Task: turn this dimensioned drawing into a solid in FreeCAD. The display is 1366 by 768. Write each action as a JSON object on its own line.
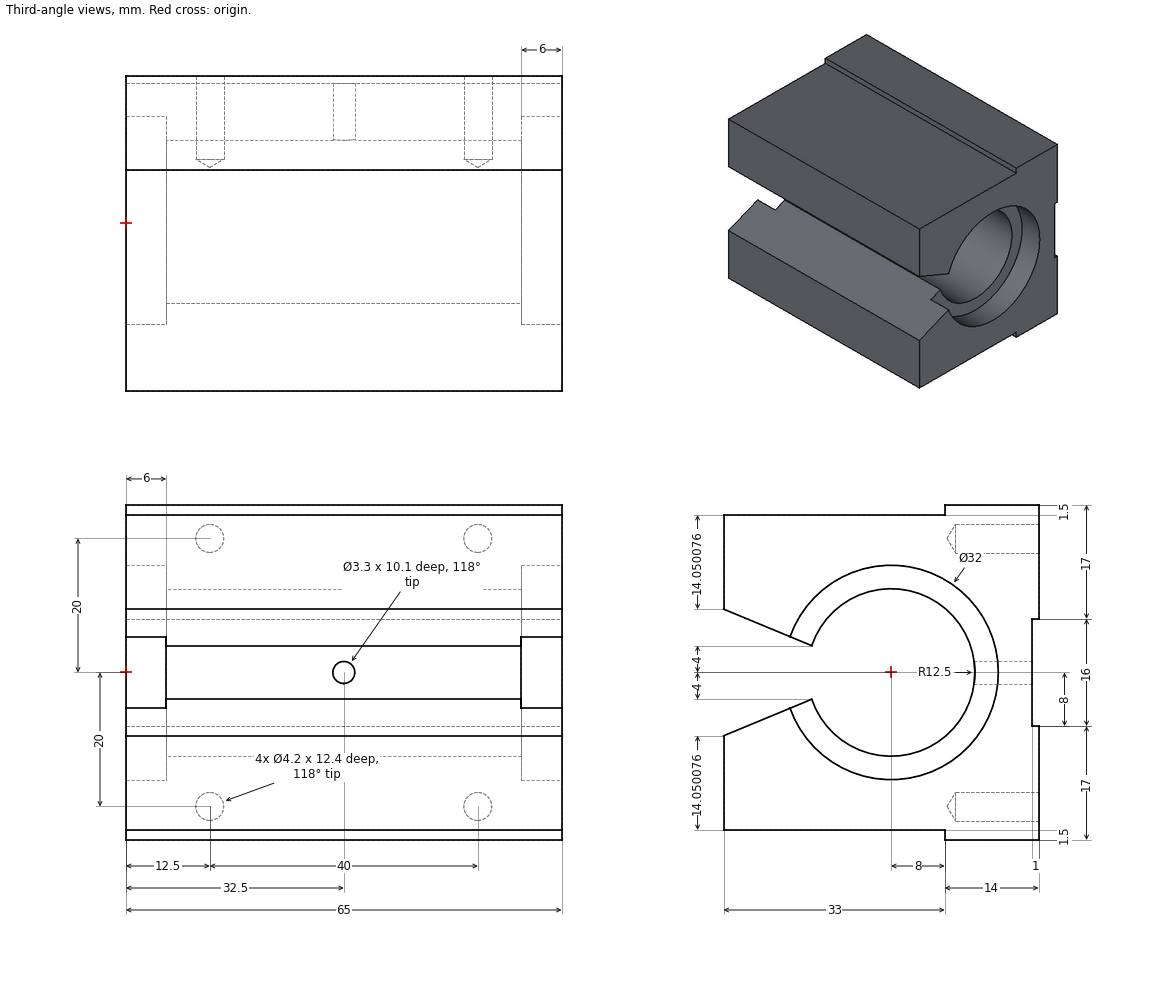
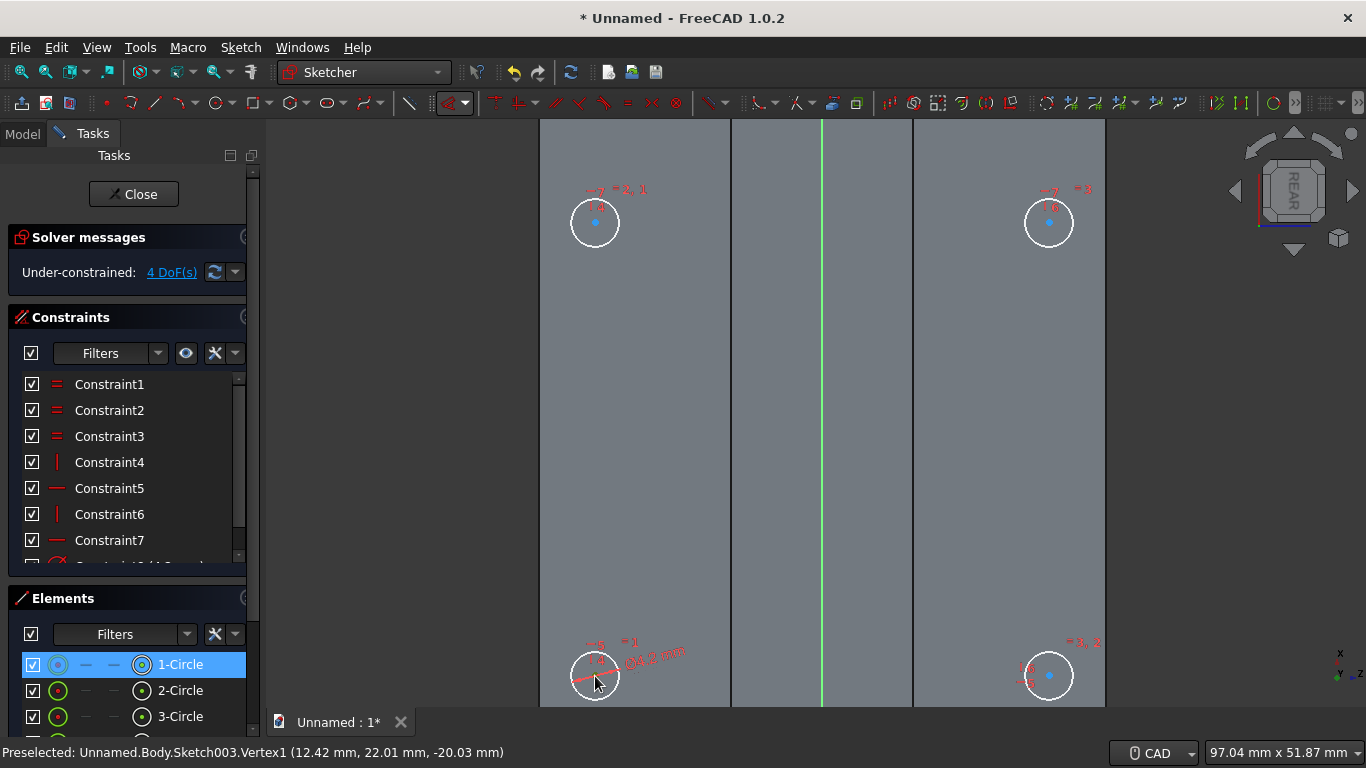
{"action": "key", "text": "l"}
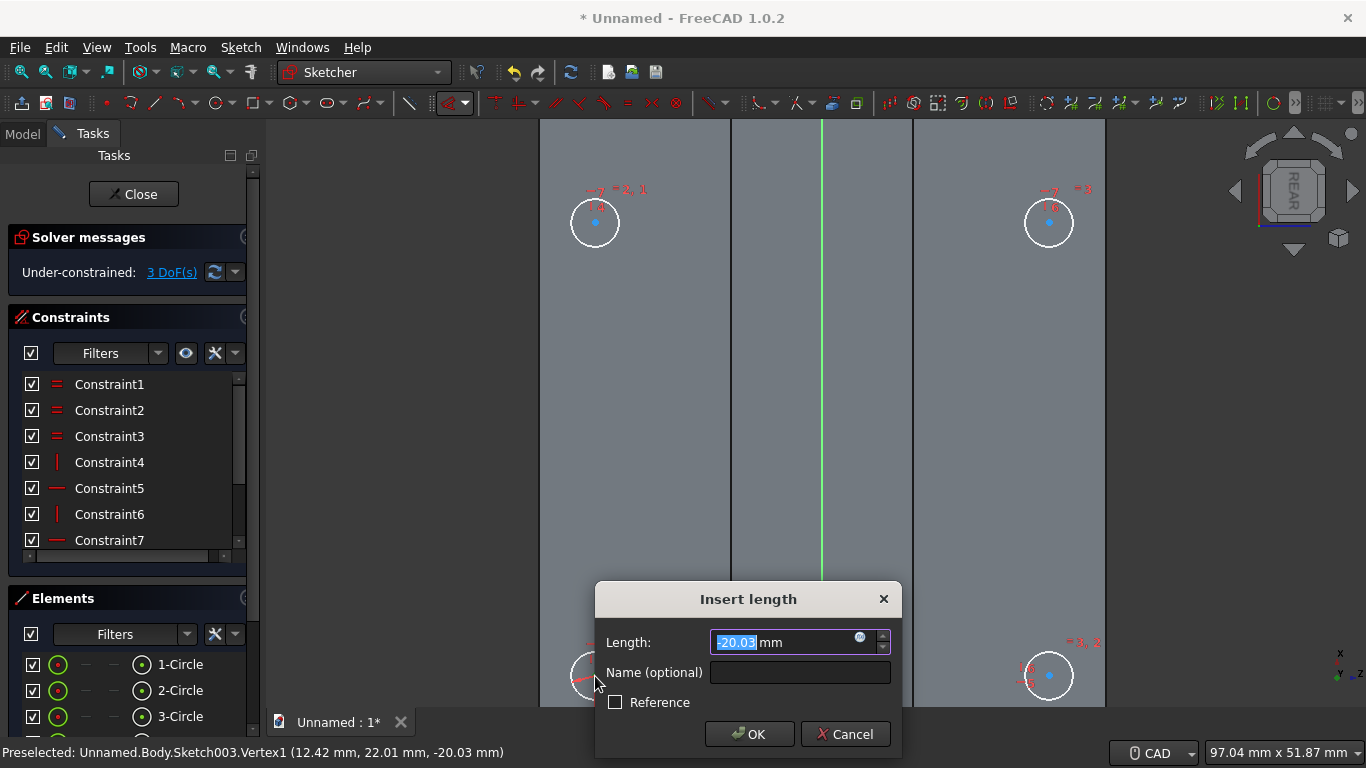
{"action": "type", "text": "-20"}
{"action": "key", "text": "Return"}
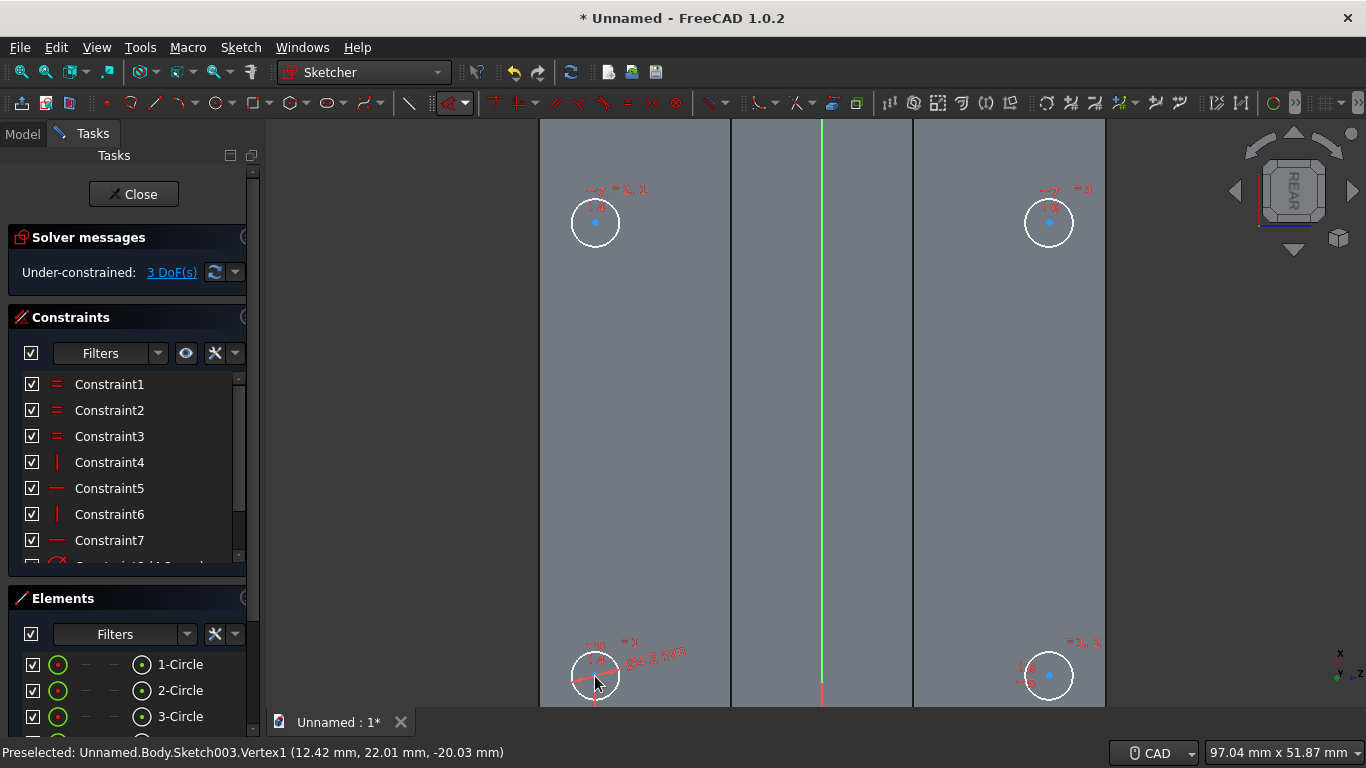
{"action": "left_click", "coordinate": [1049, 676]}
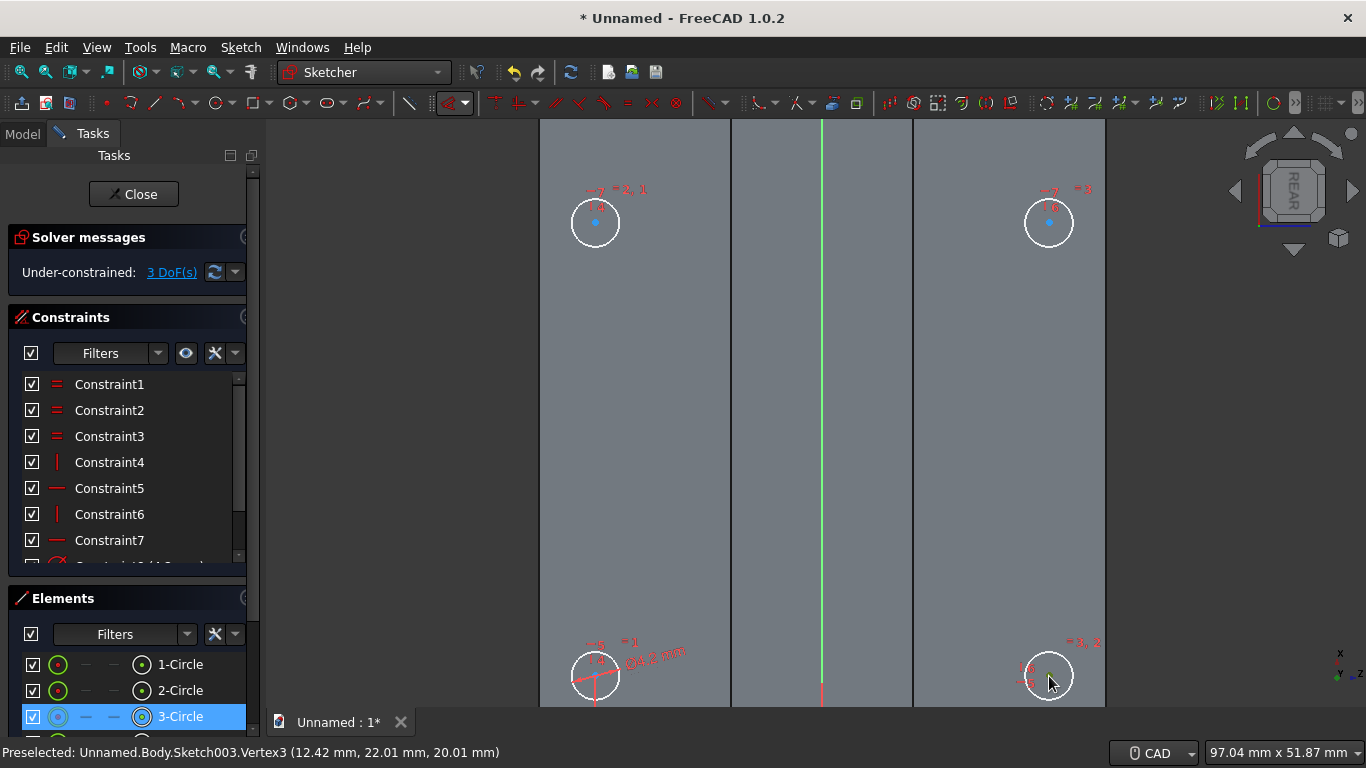
{"action": "left_click", "coordinate": [468, 104]}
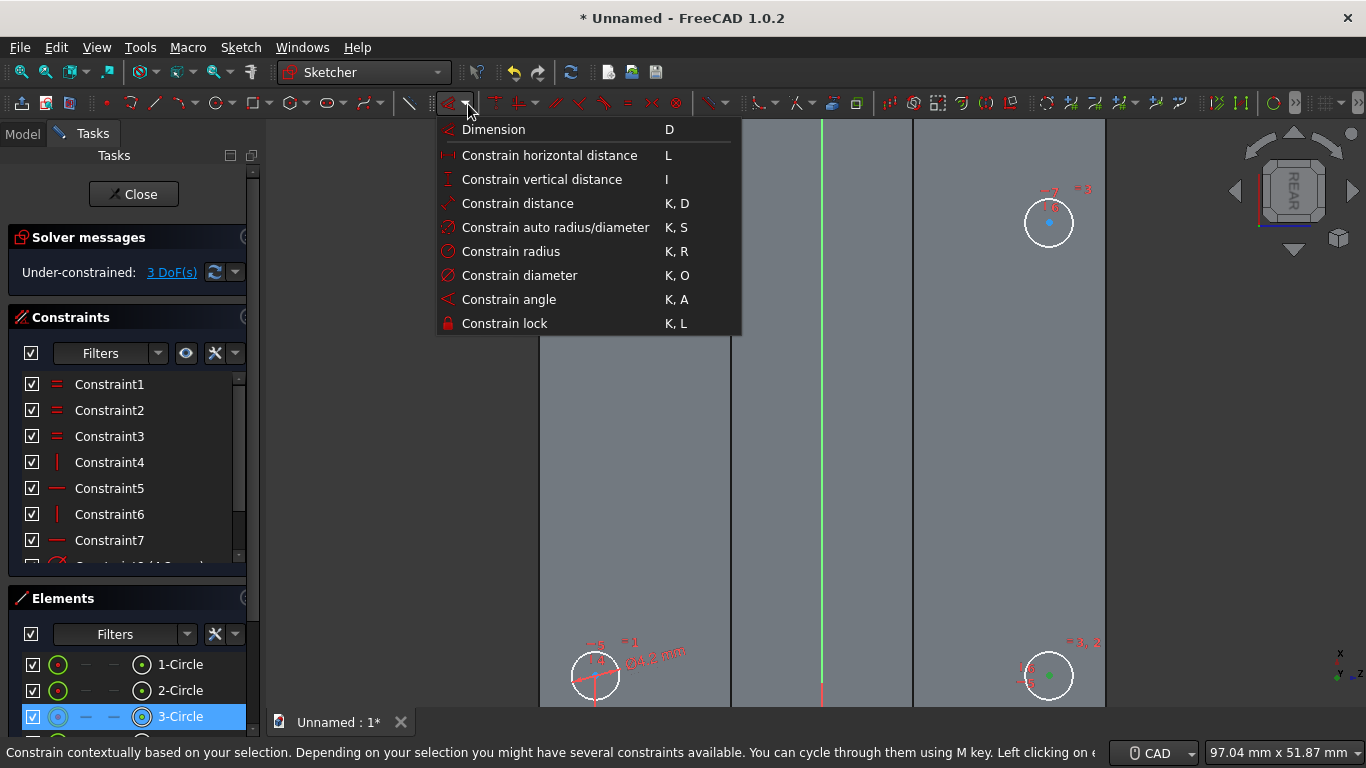
{"action": "left_click", "coordinate": [589, 155]}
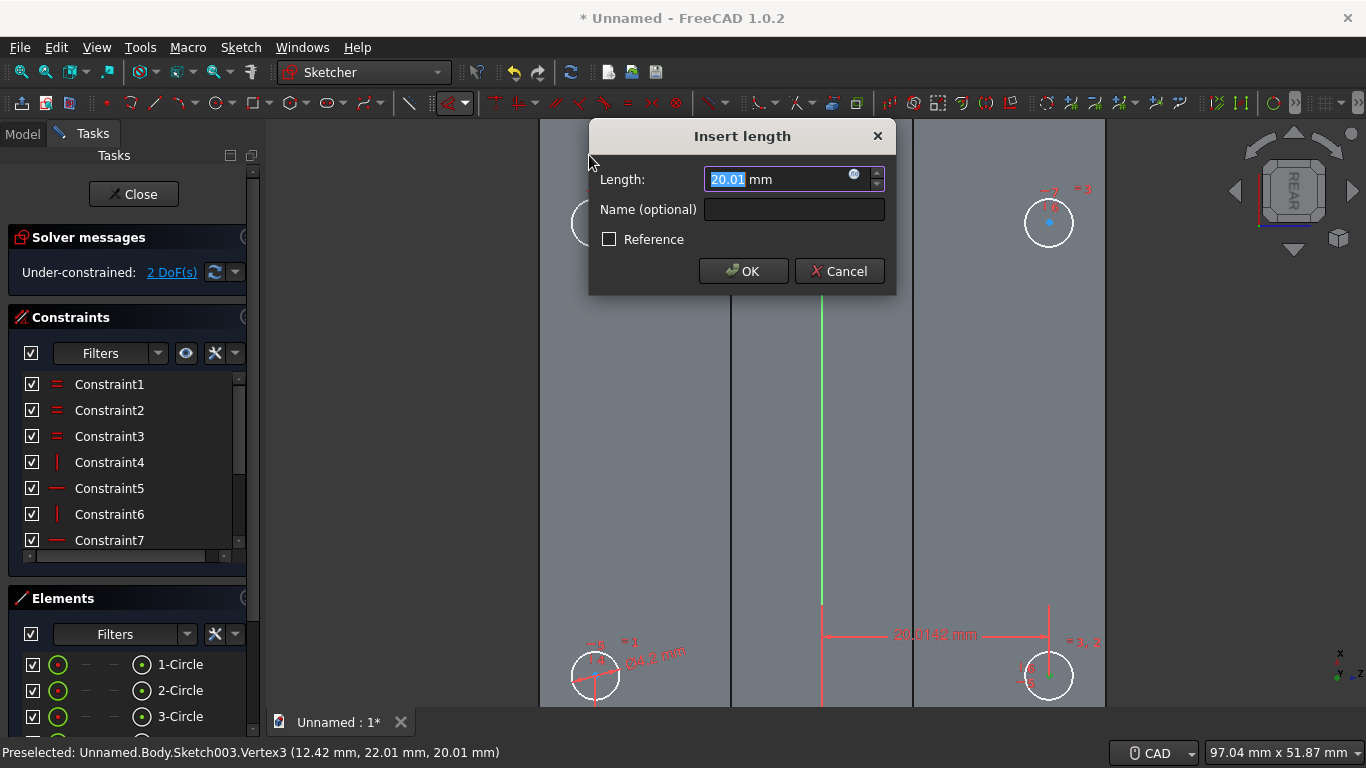
{"action": "type", "text": "20"}
{"action": "key", "text": "Return"}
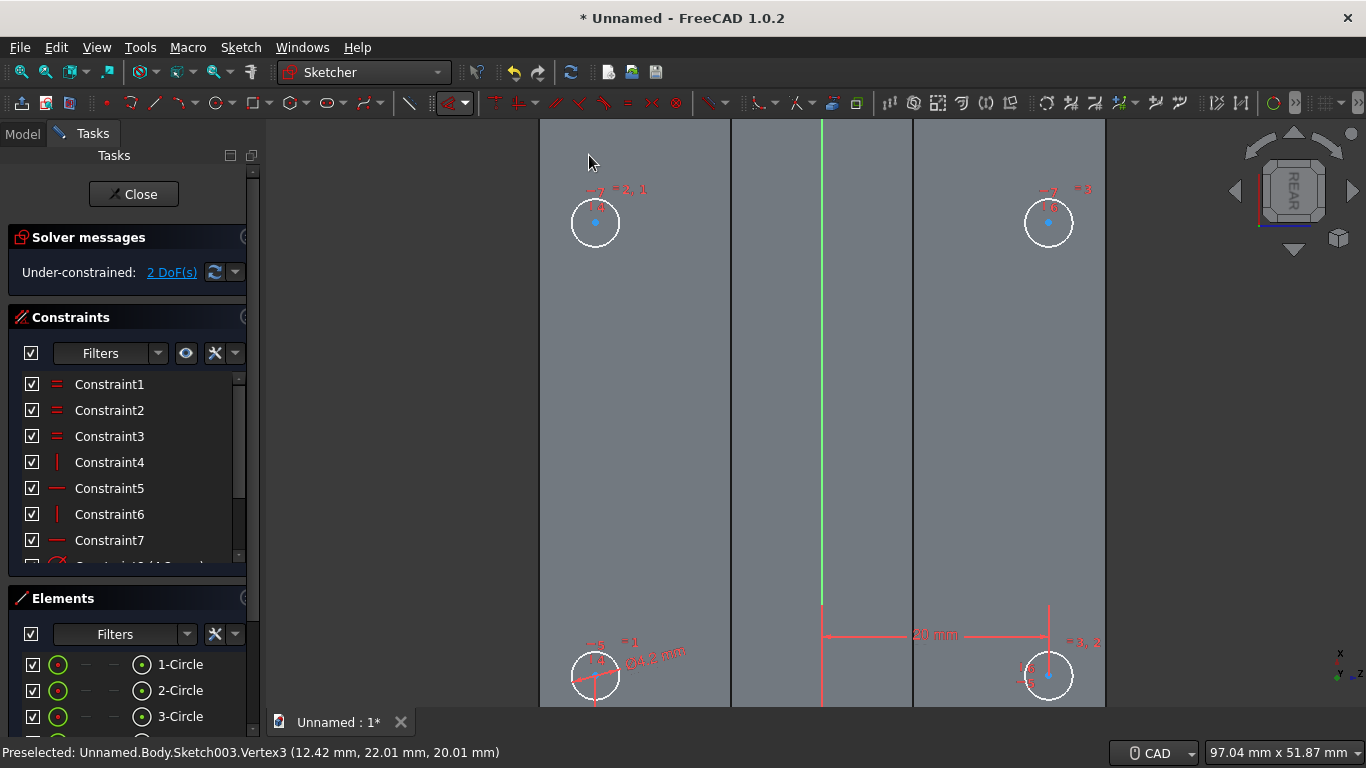
{"action": "left_click", "coordinate": [595, 676]}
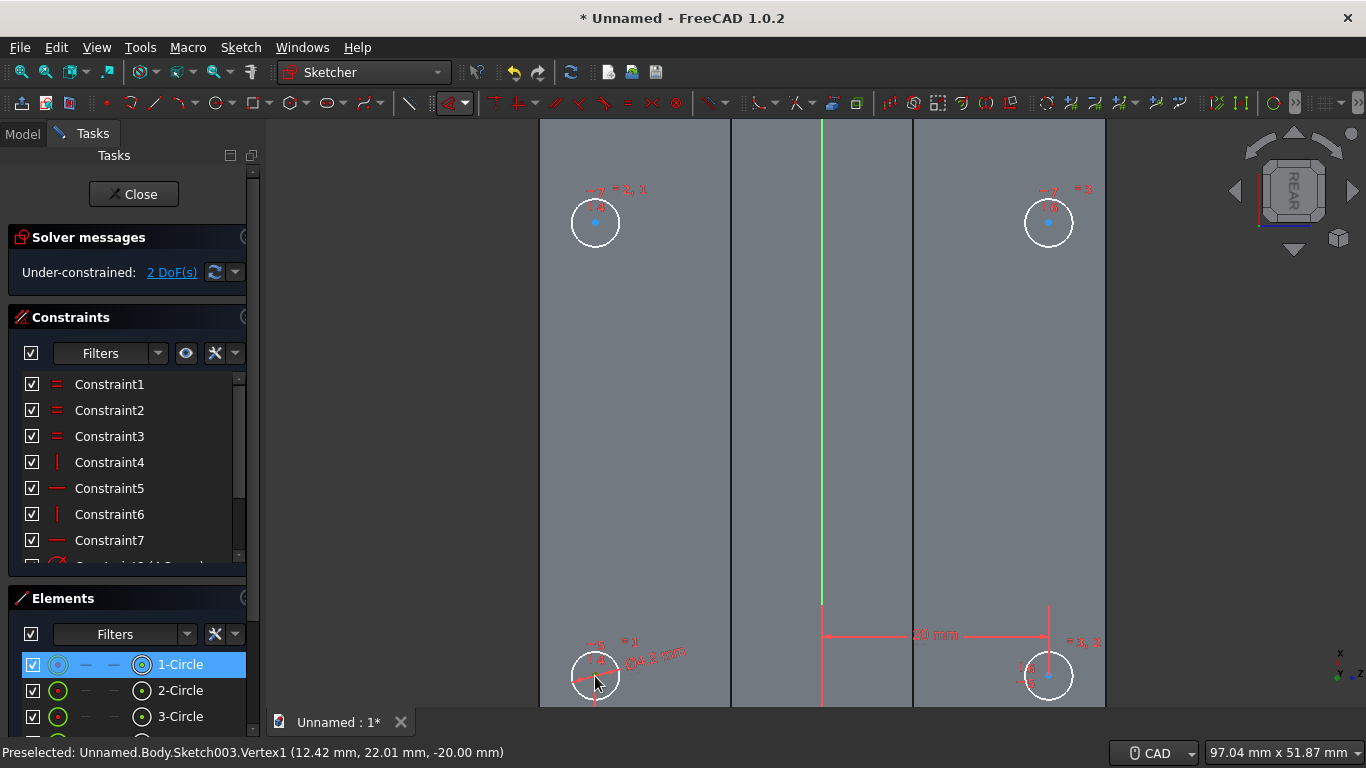
{"action": "left_click", "coordinate": [595, 223]}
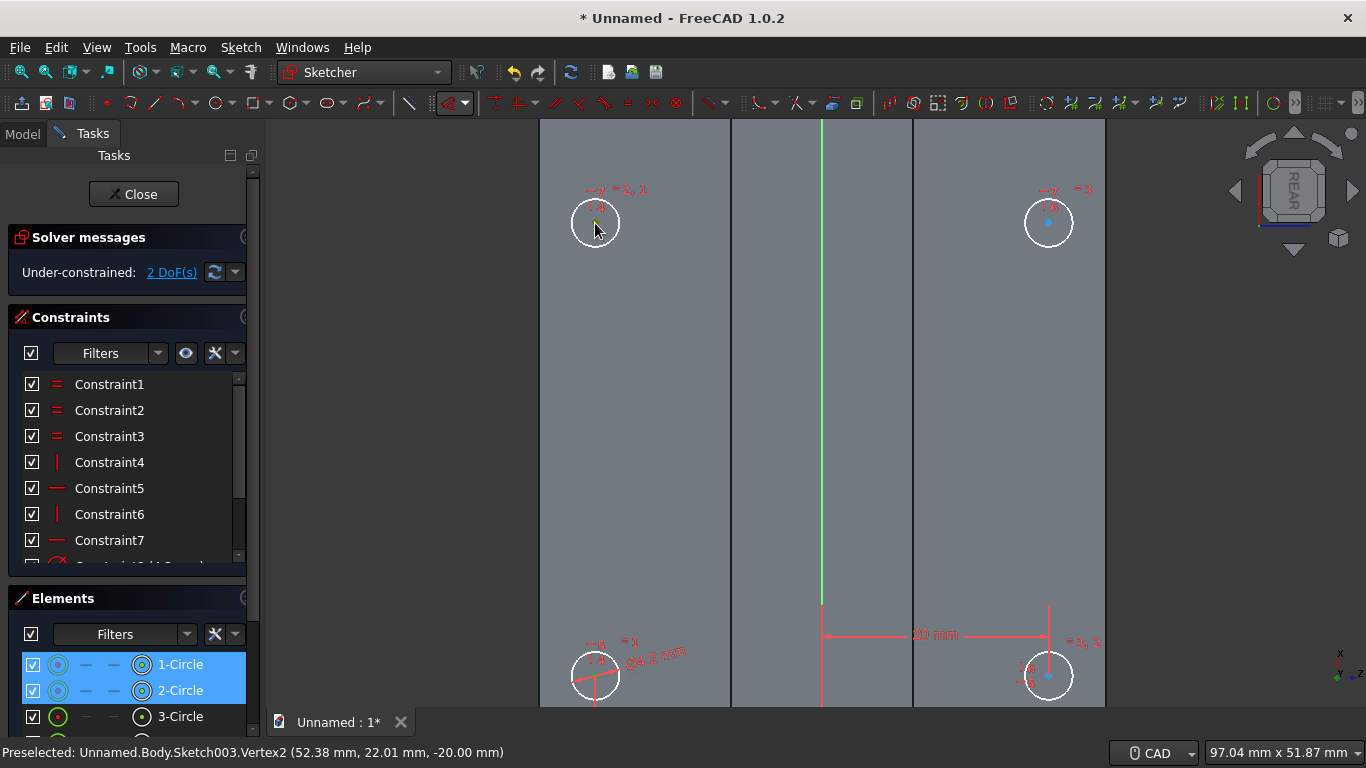
{"action": "key", "text": "i"}